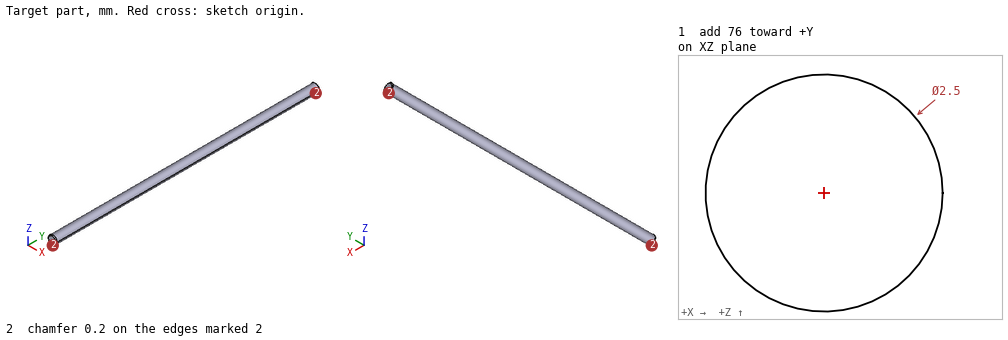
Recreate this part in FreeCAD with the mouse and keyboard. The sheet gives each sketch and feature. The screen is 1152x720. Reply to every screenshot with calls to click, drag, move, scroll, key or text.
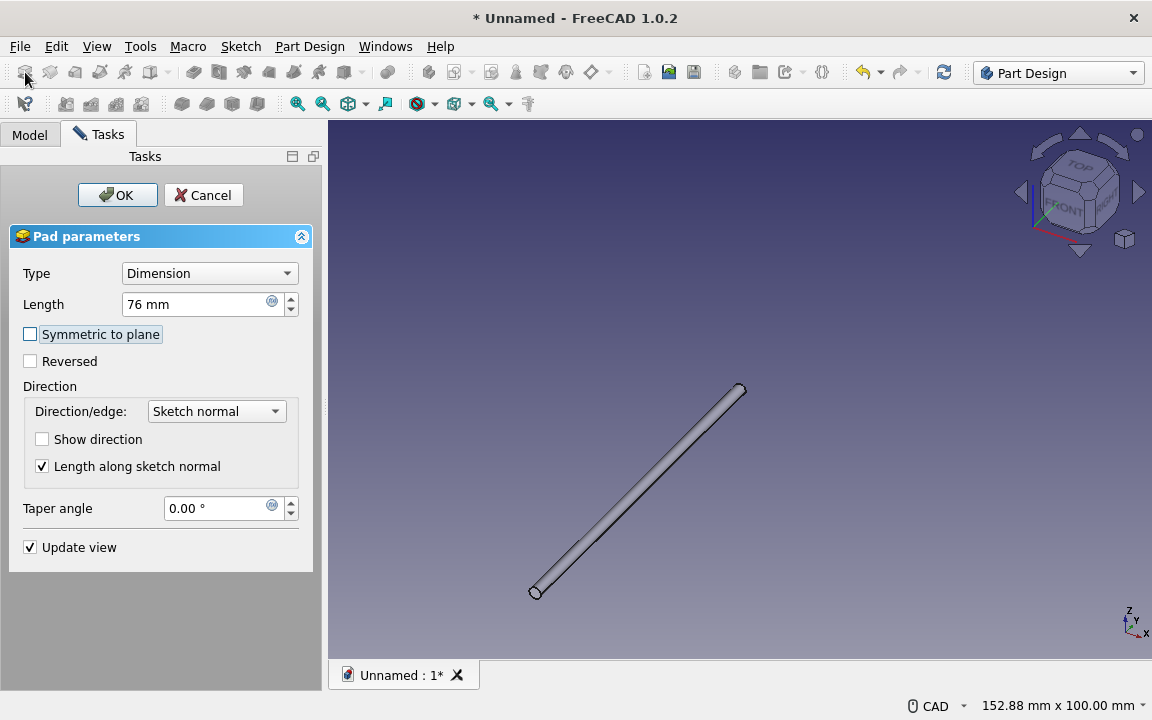
click(31, 361)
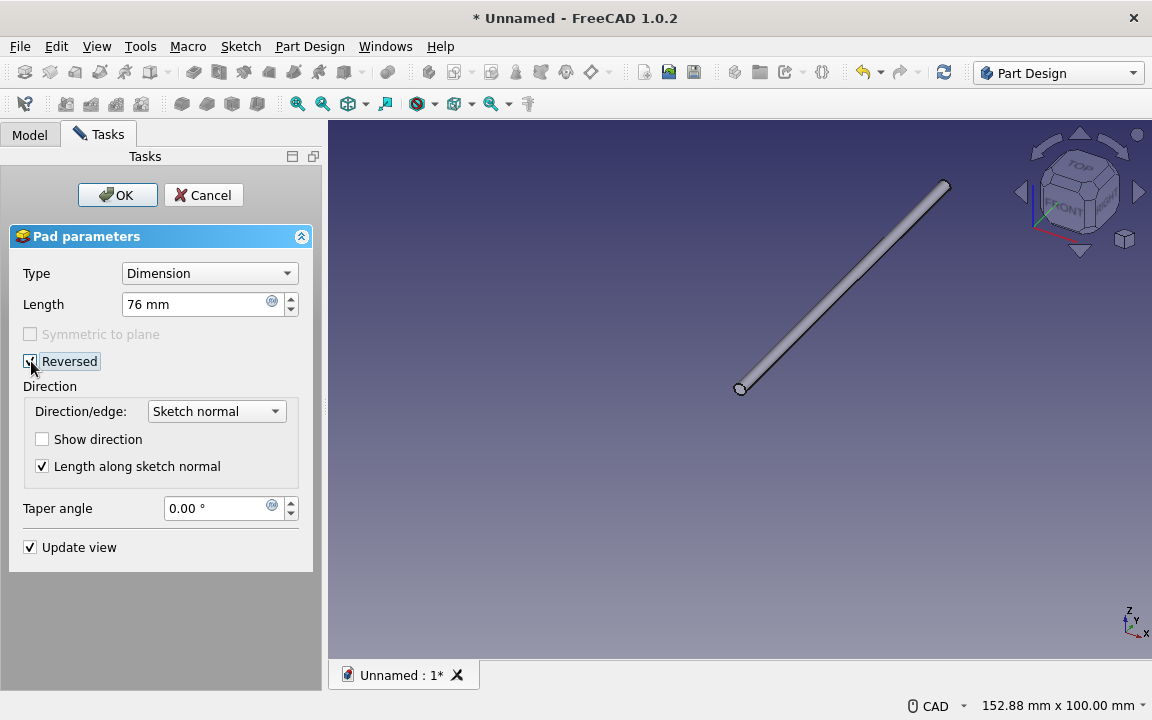
click(118, 195)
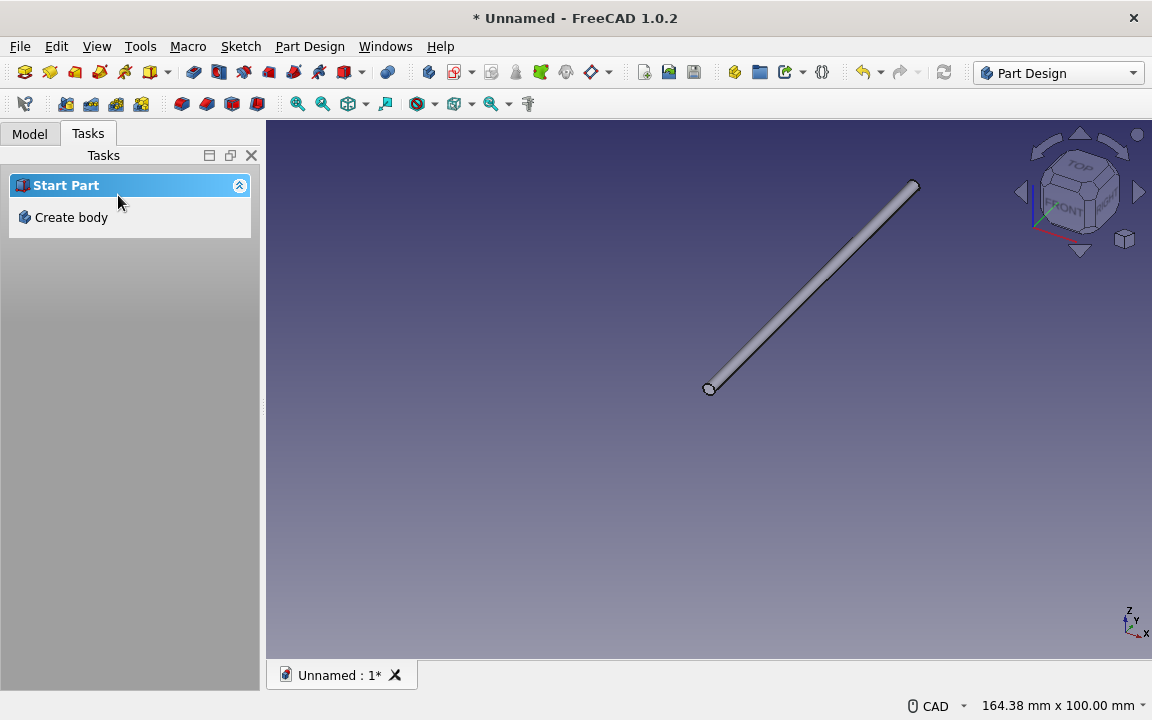
click(298, 104)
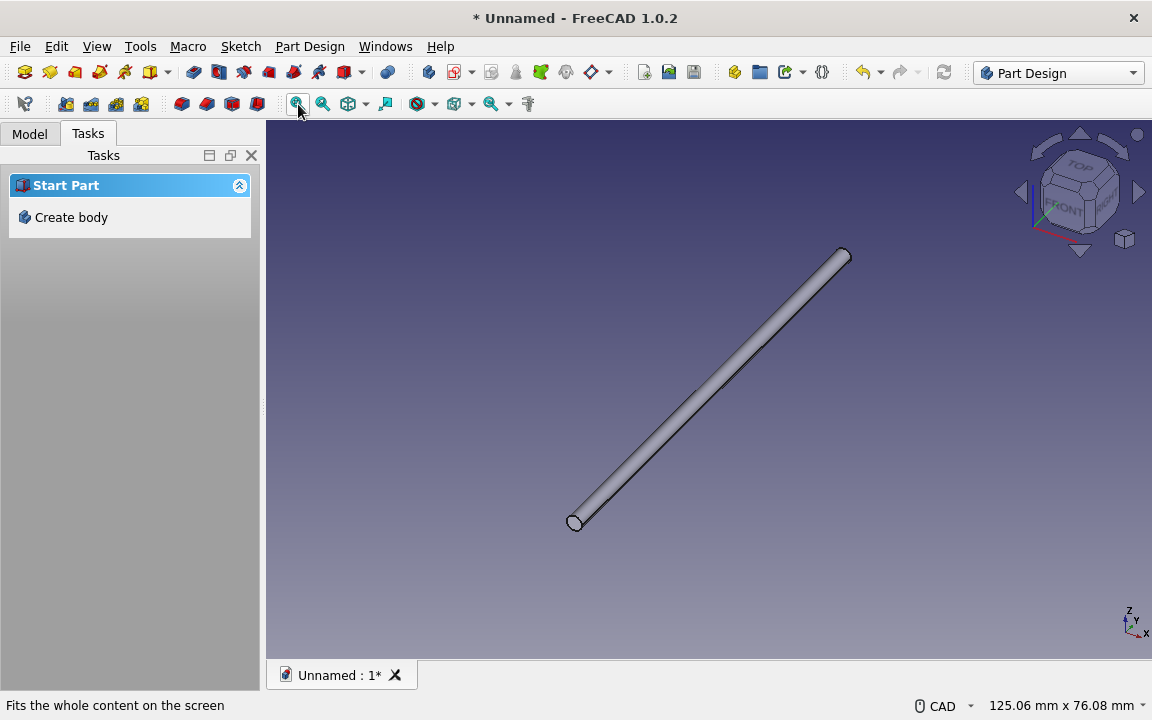
click(567, 520)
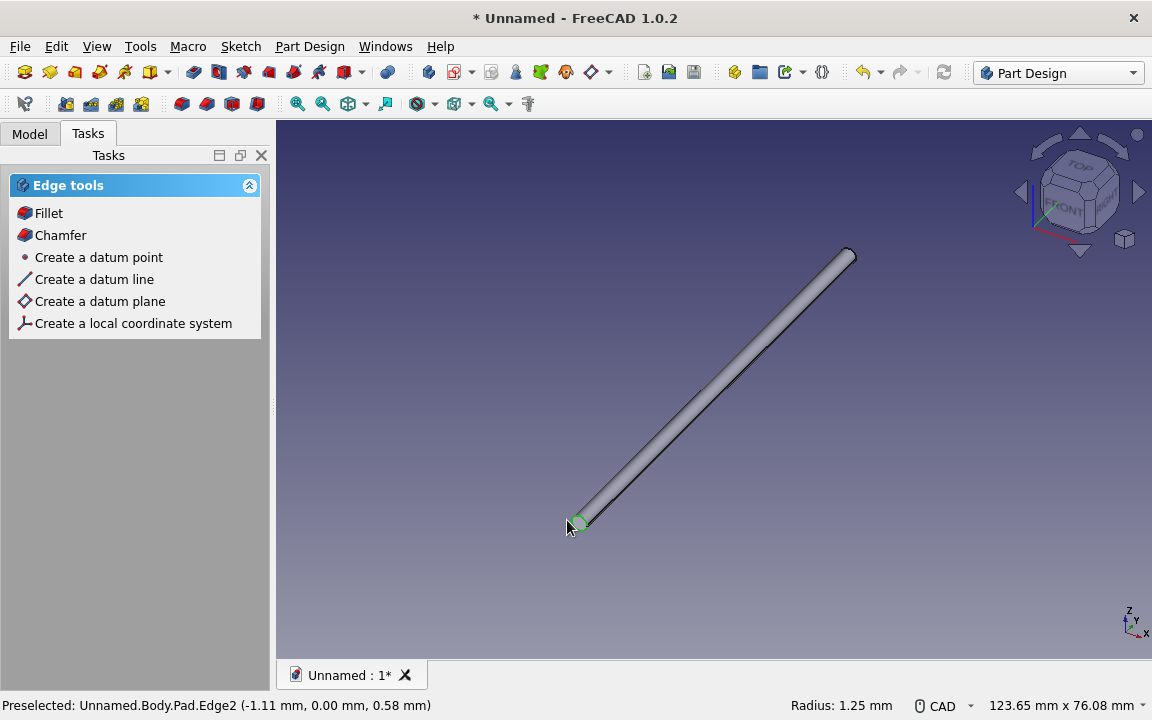
click(846, 247, ctrl)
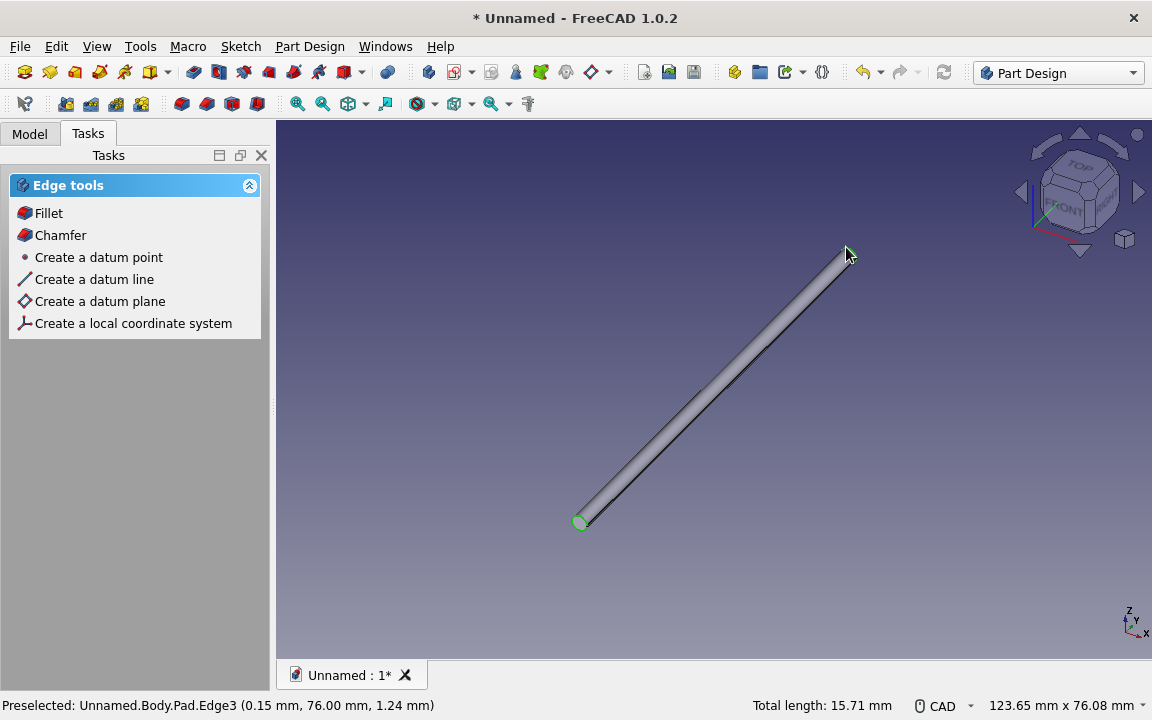
click(207, 104)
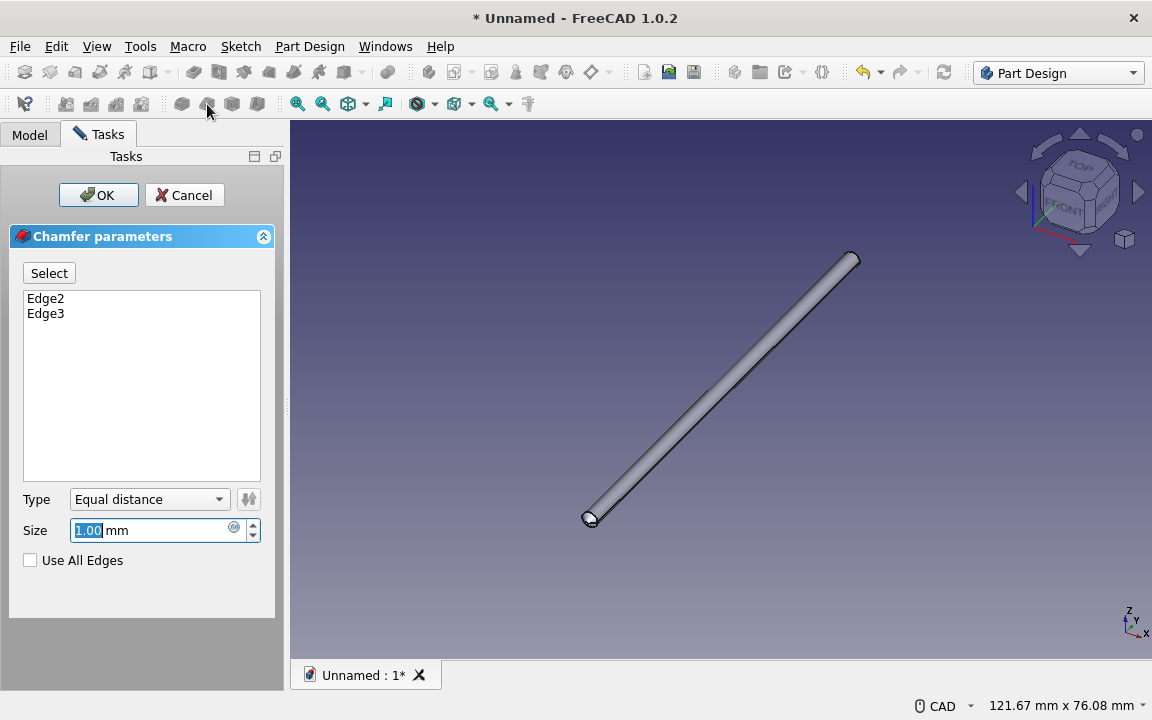
text(0.2)
key(Tab)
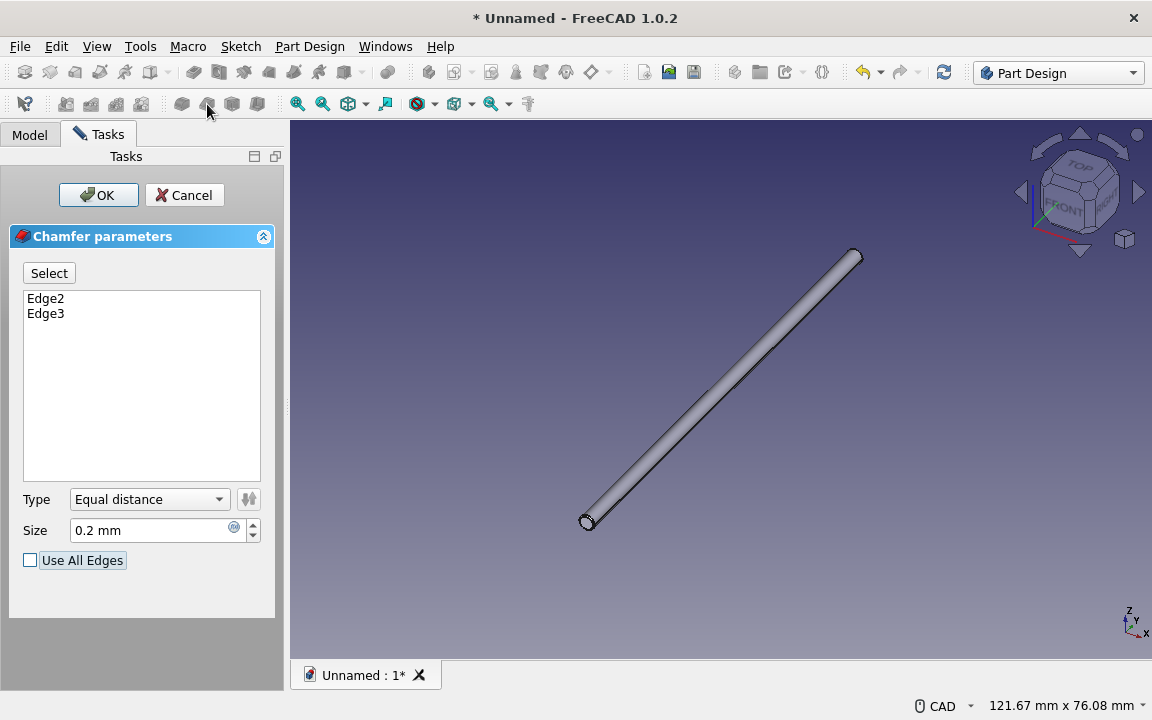
click(99, 195)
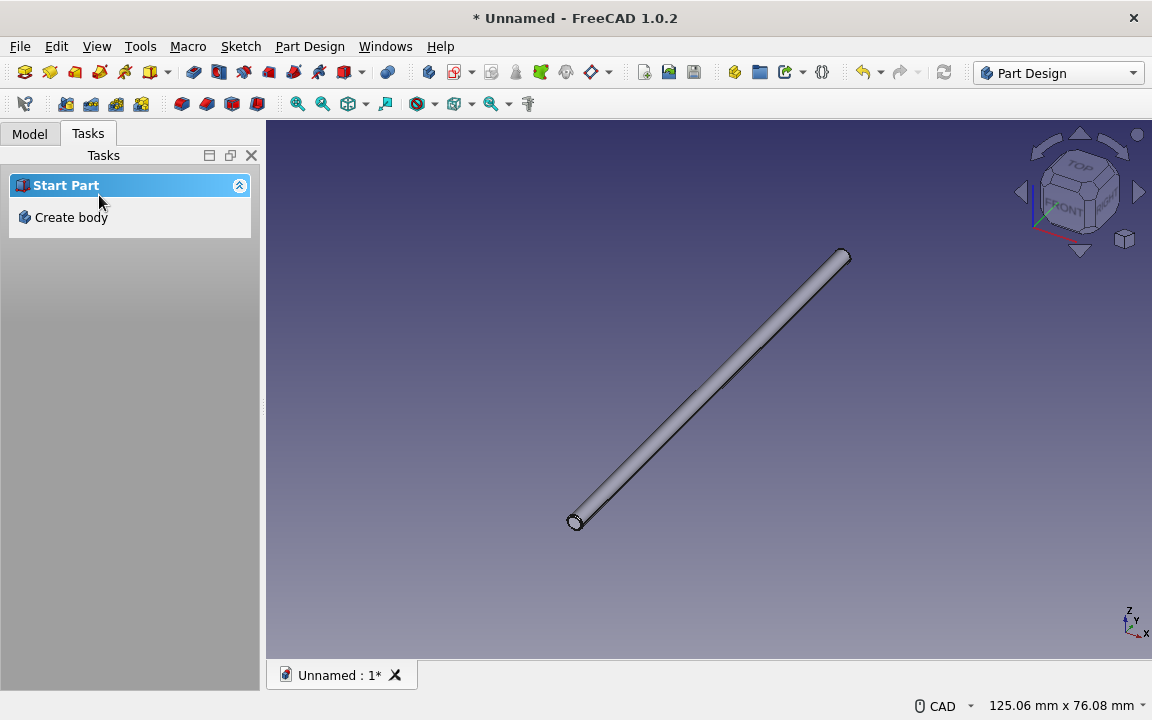
key(0)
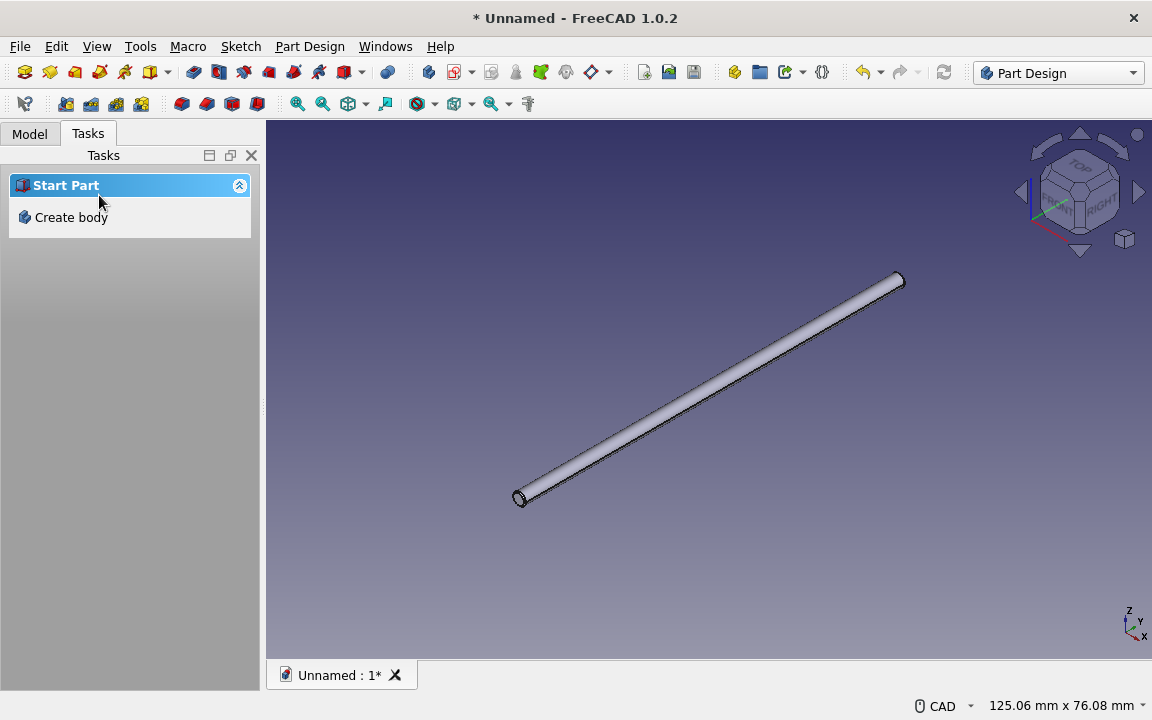
click(298, 104)